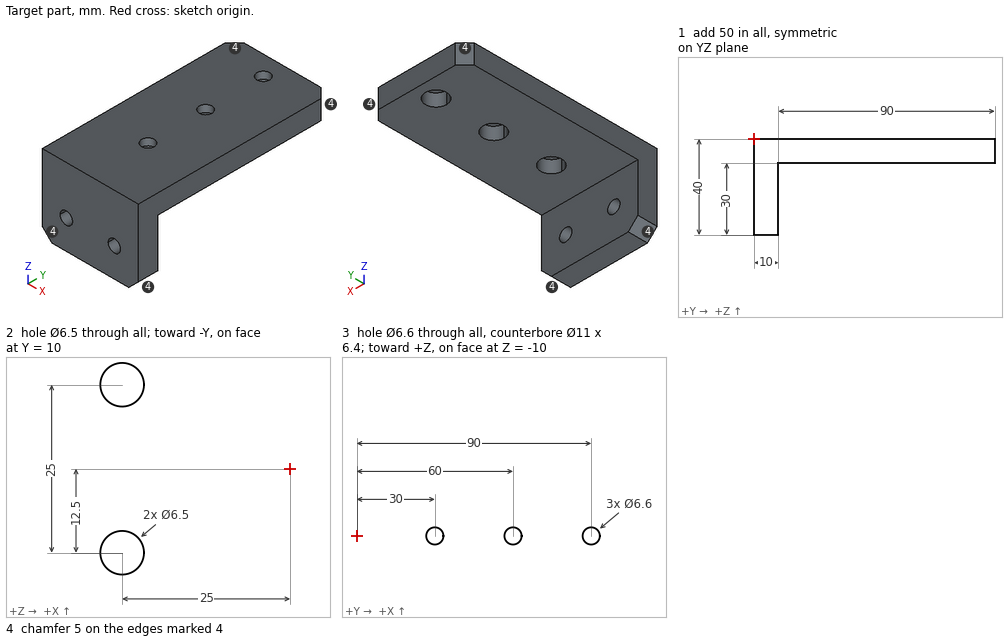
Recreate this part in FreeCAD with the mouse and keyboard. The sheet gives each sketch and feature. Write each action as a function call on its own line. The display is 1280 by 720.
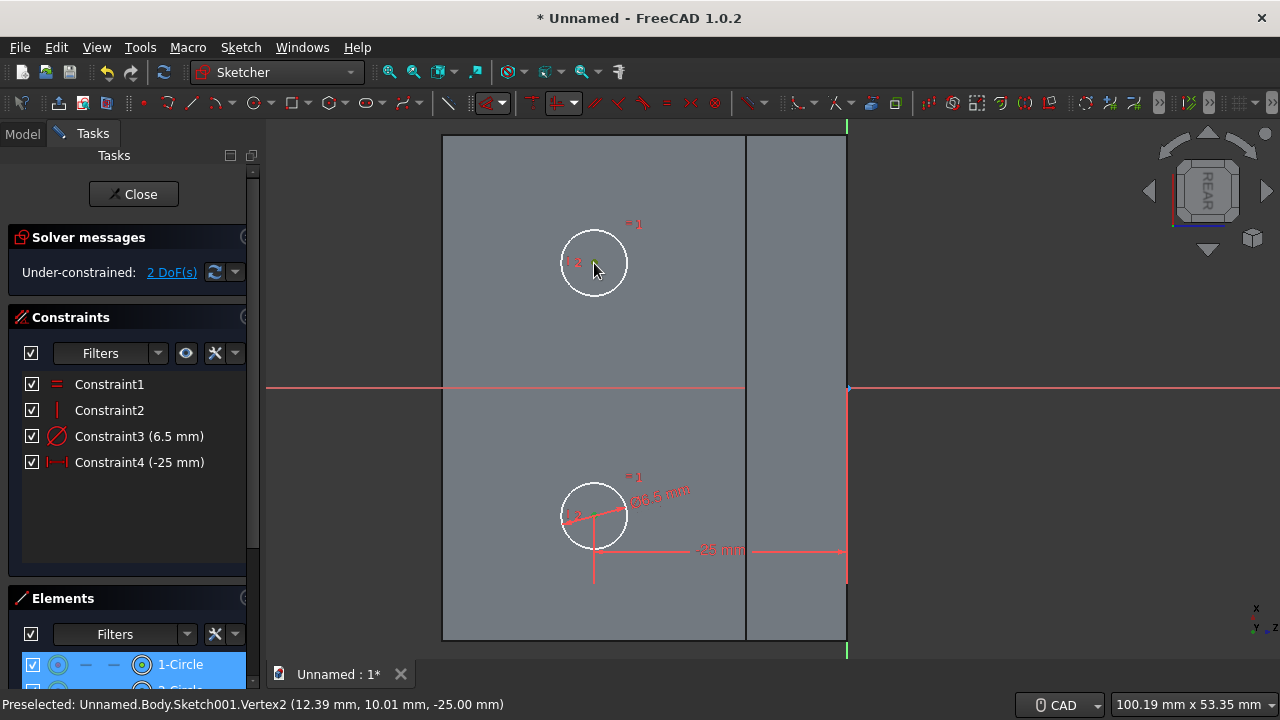
click(504, 104)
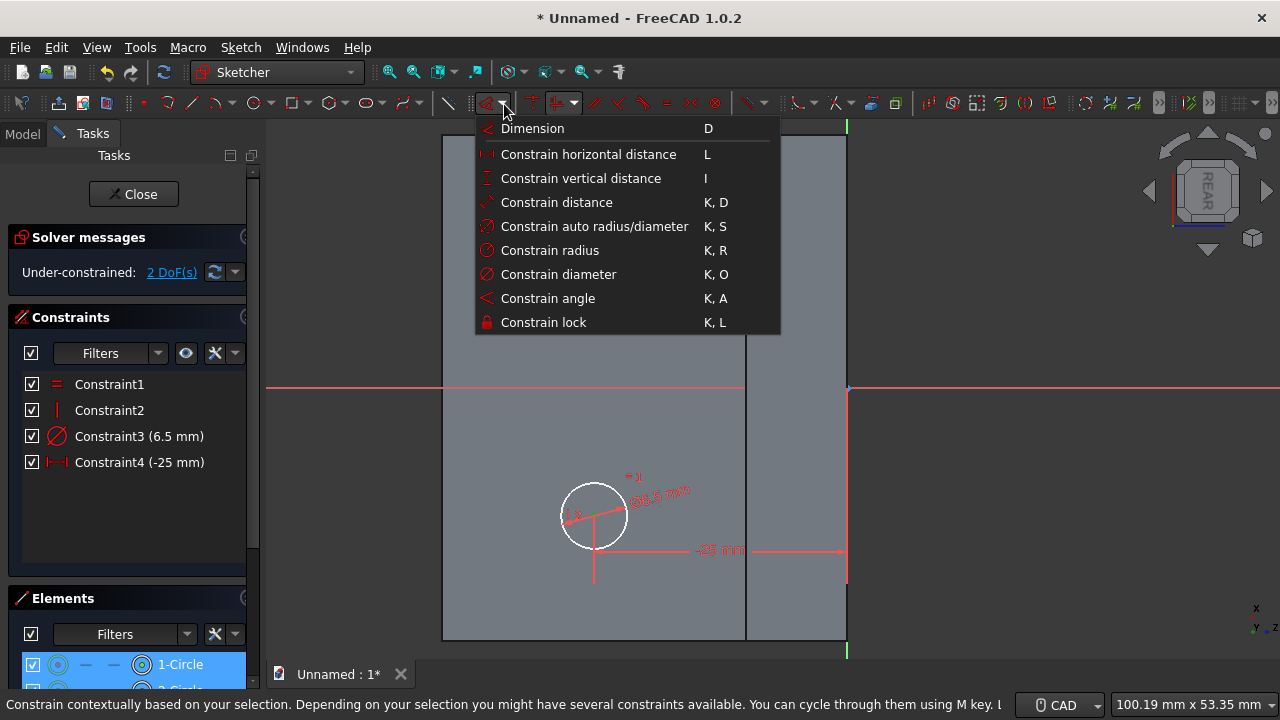
click(628, 178)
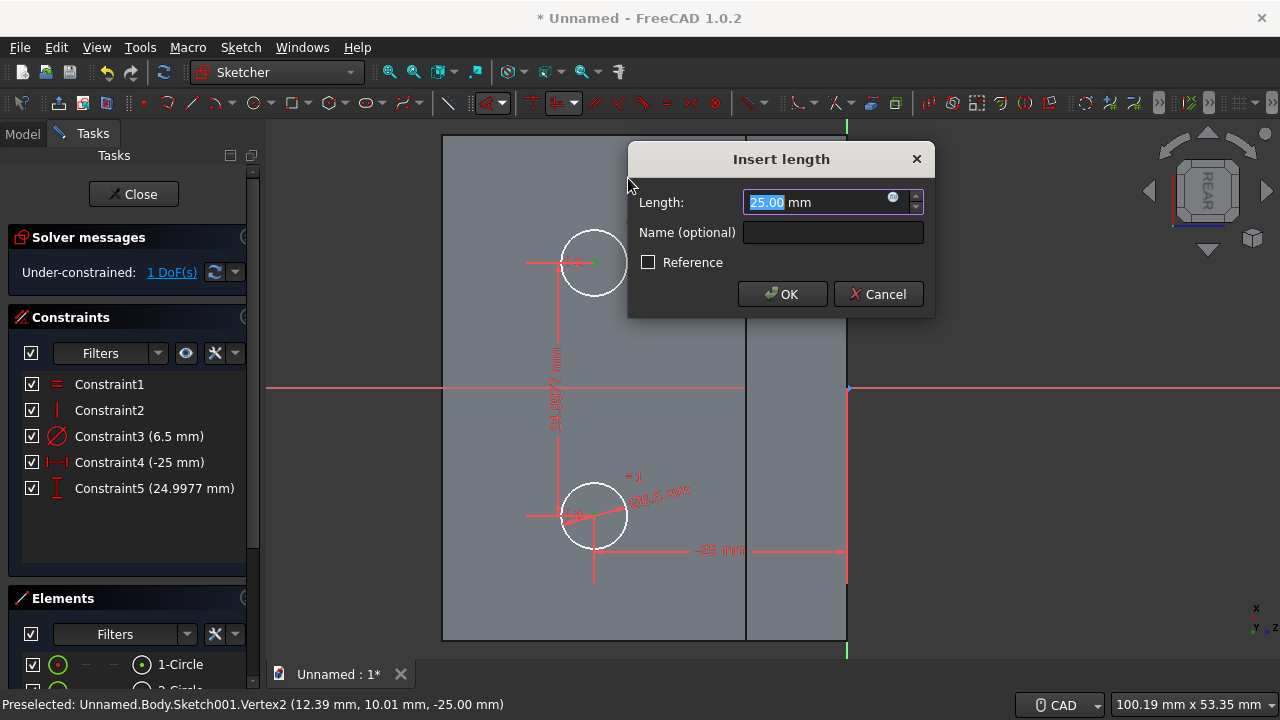
text(25)
key(Return)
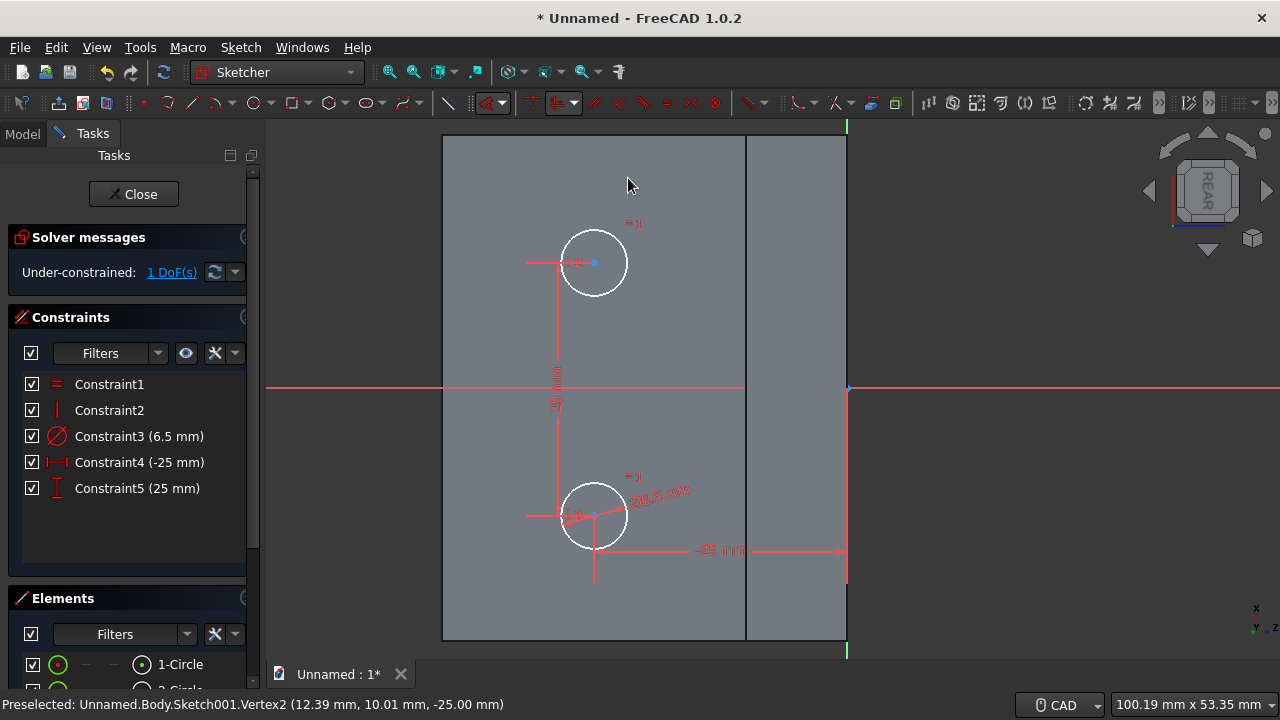
click(594, 516)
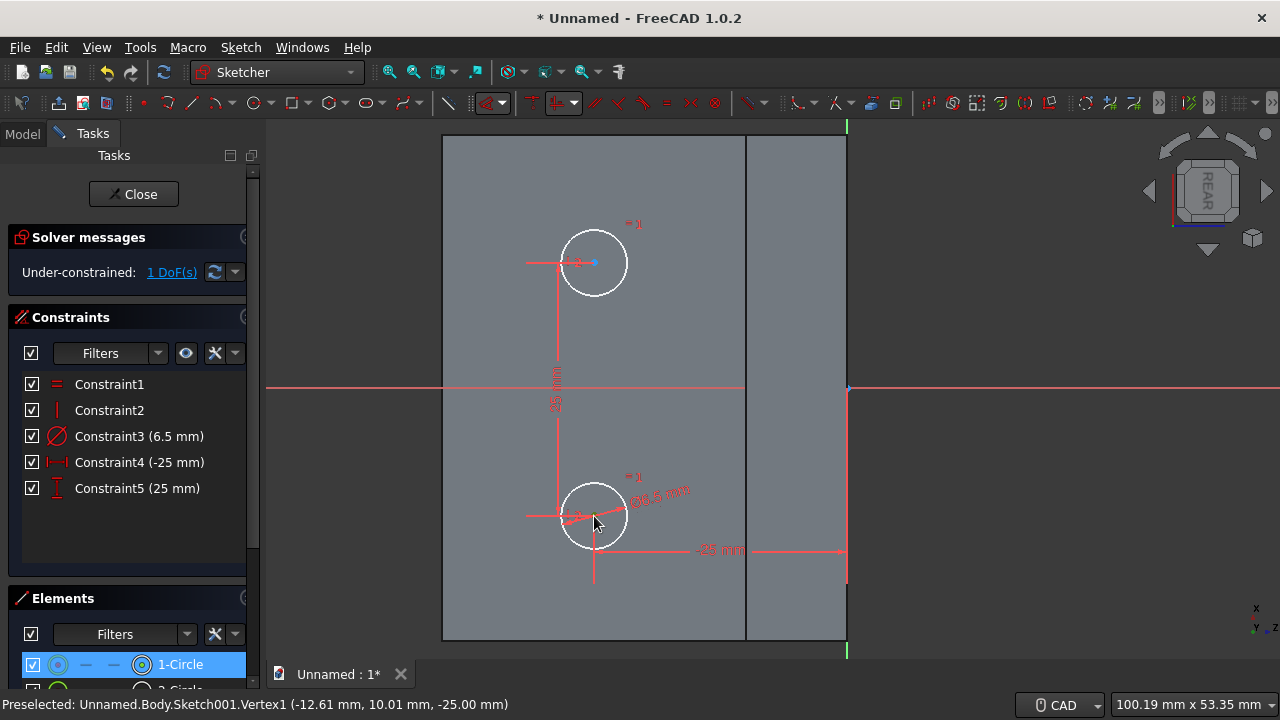
key(i)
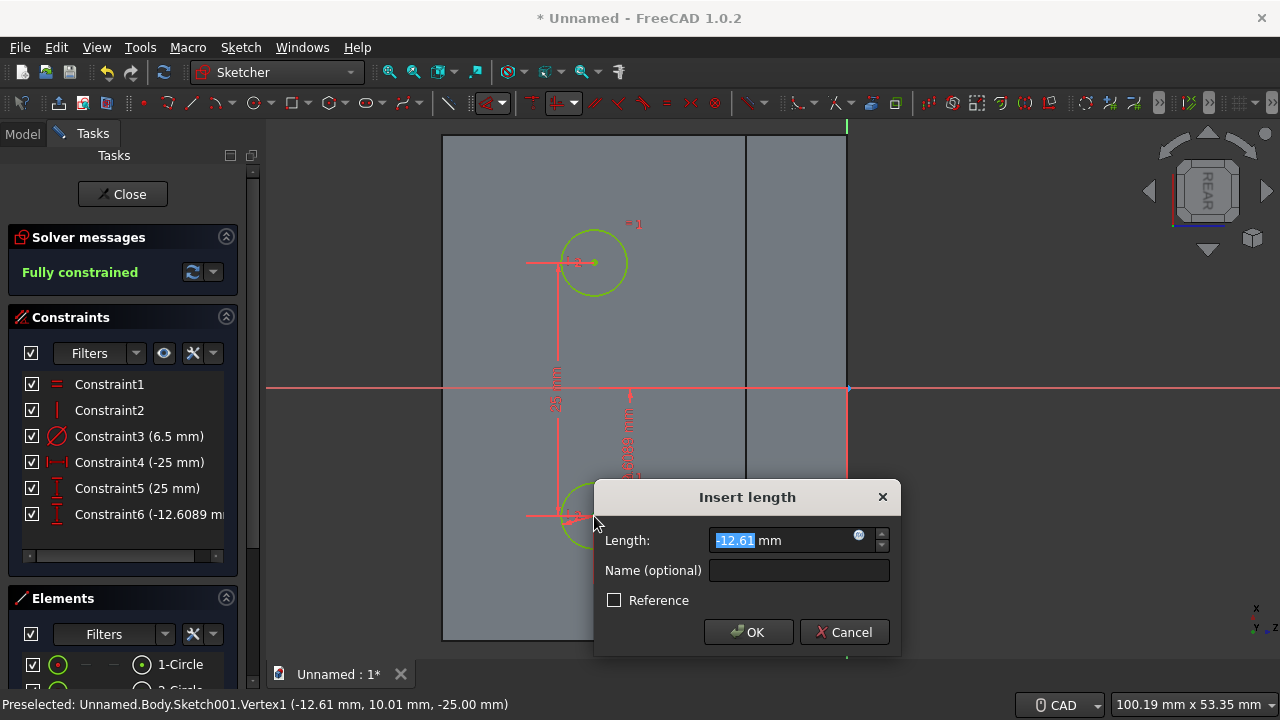
text(-12.5)
key(Return)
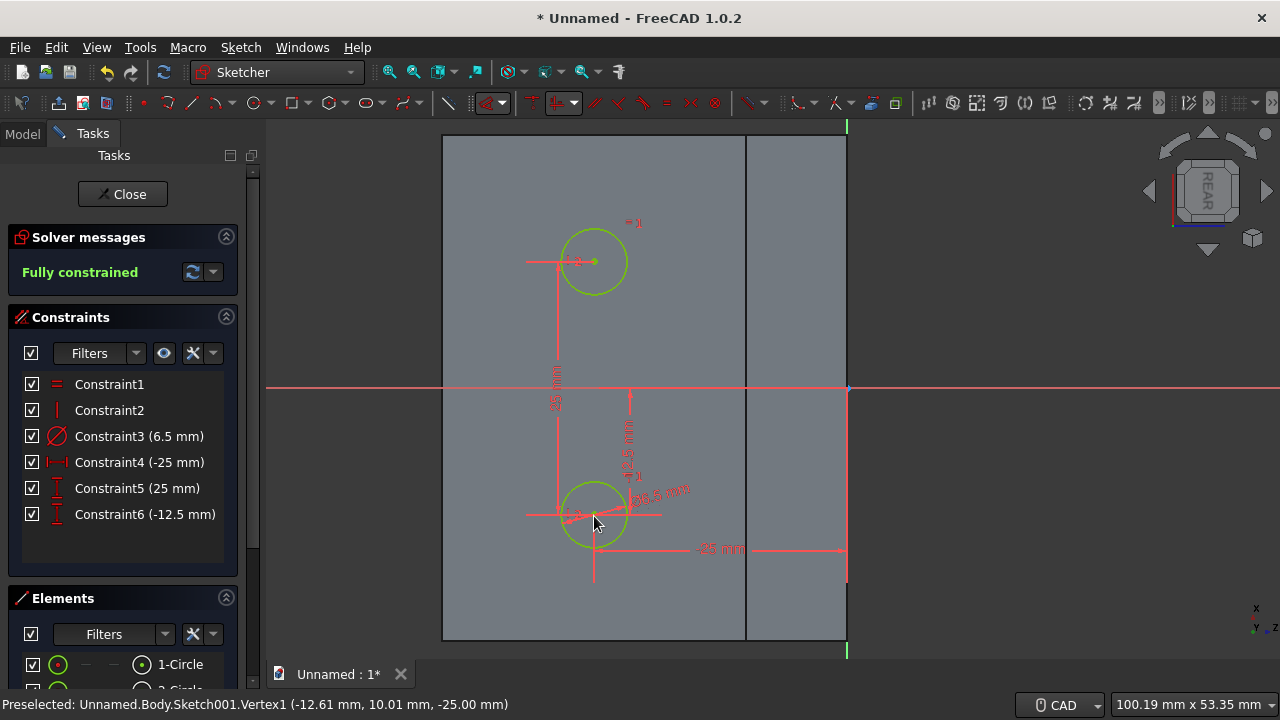
click(123, 194)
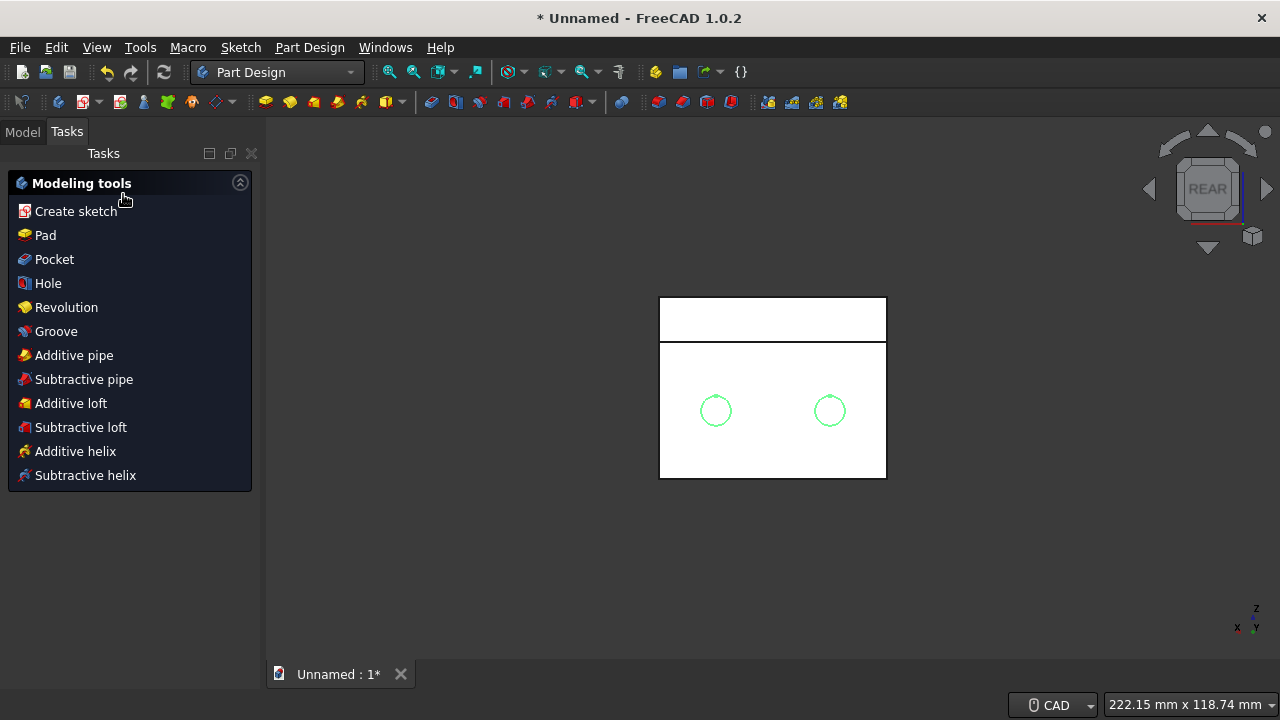
click(456, 102)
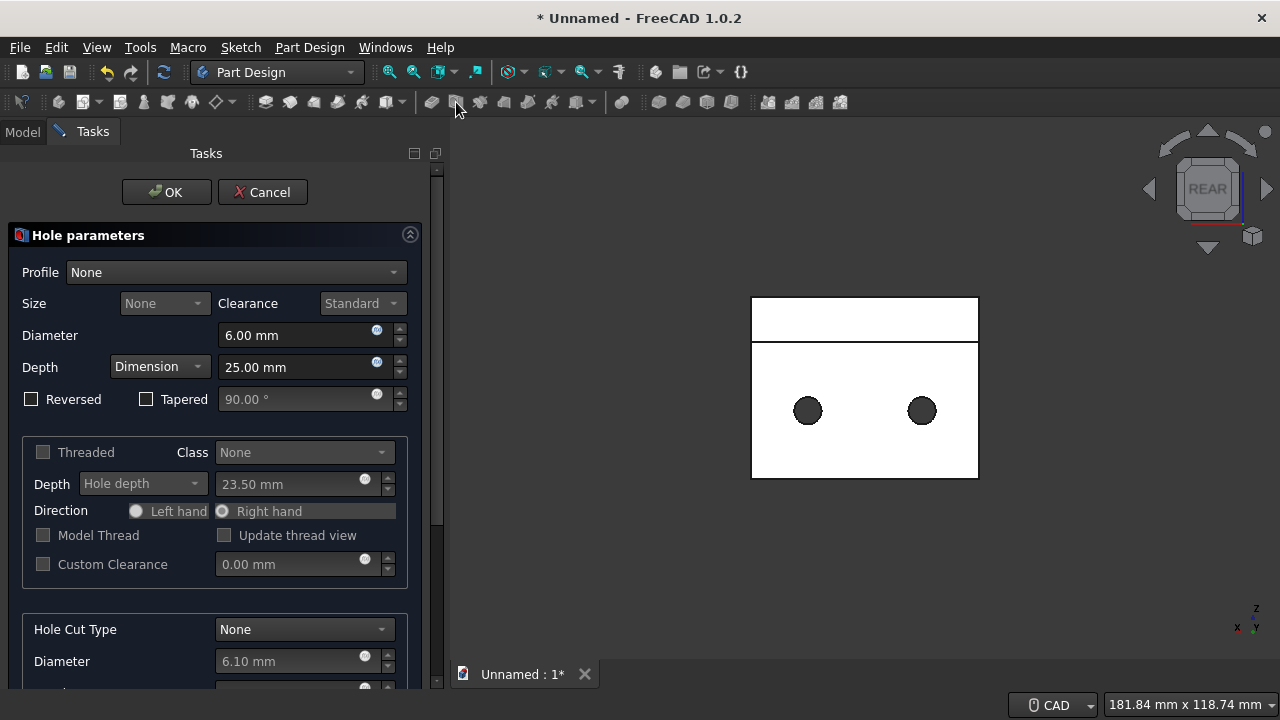
triple_click(305, 335)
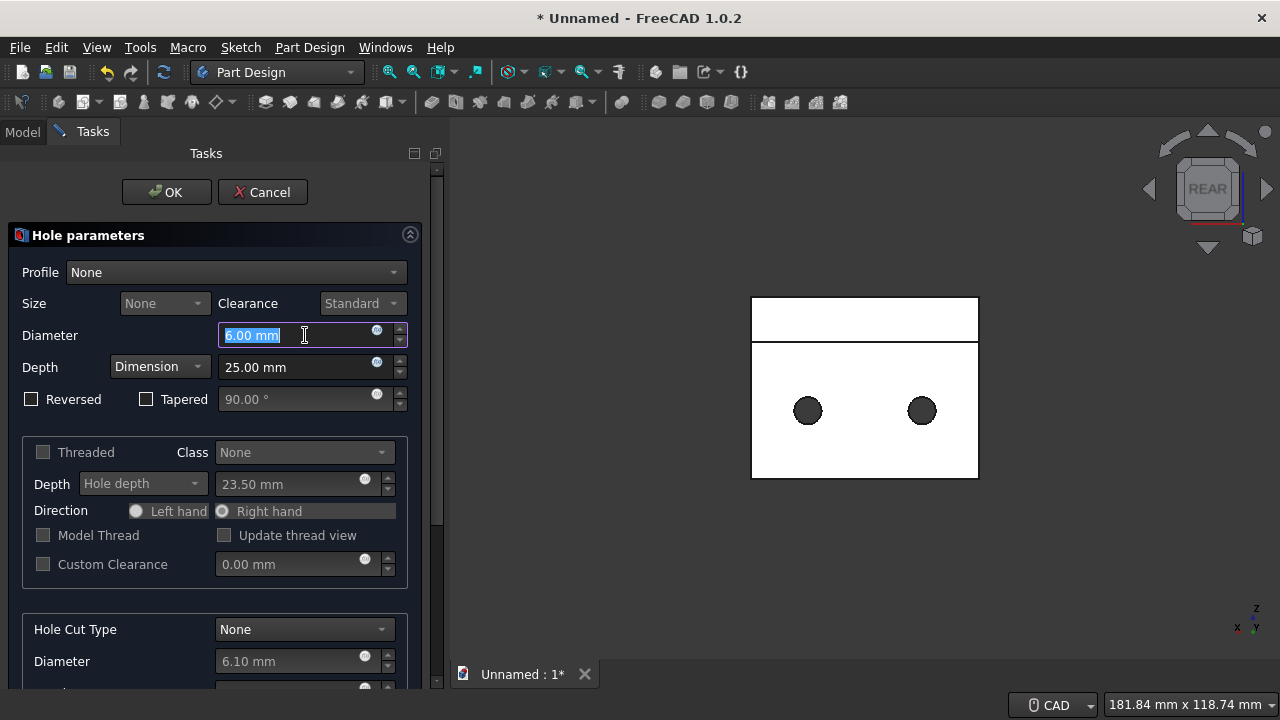
text(6.5)
key(Tab)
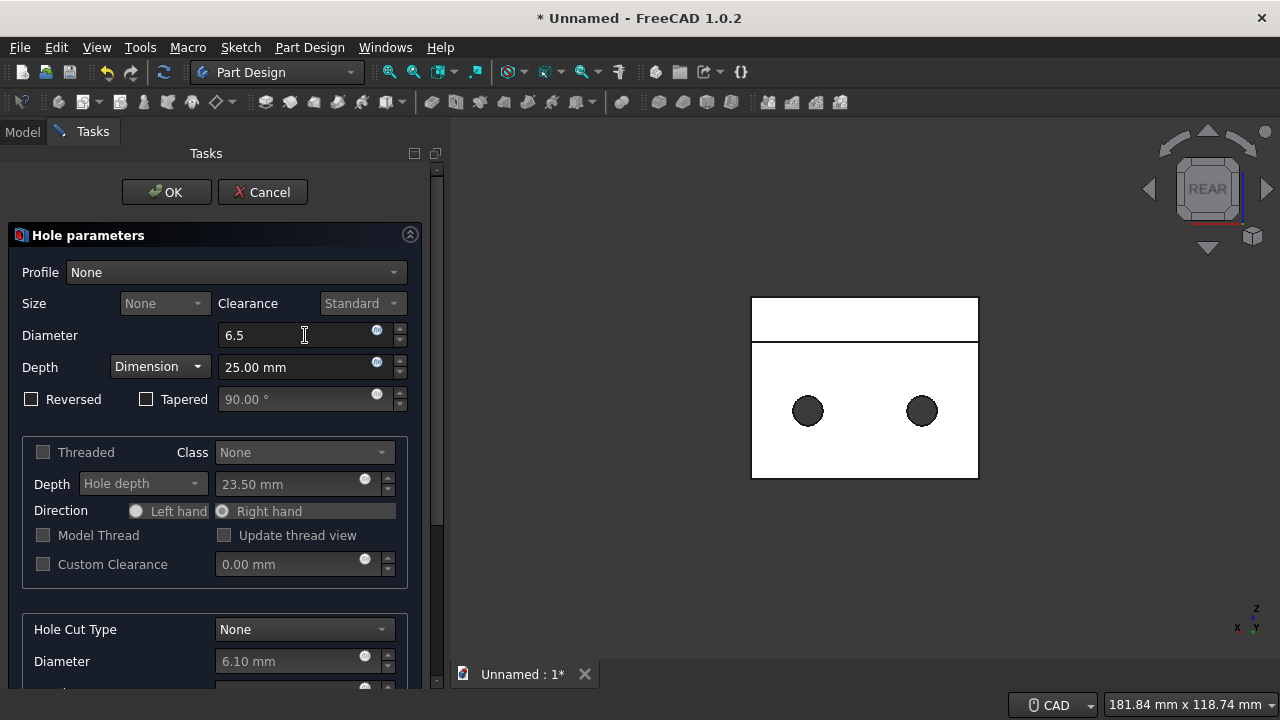
click(161, 366)